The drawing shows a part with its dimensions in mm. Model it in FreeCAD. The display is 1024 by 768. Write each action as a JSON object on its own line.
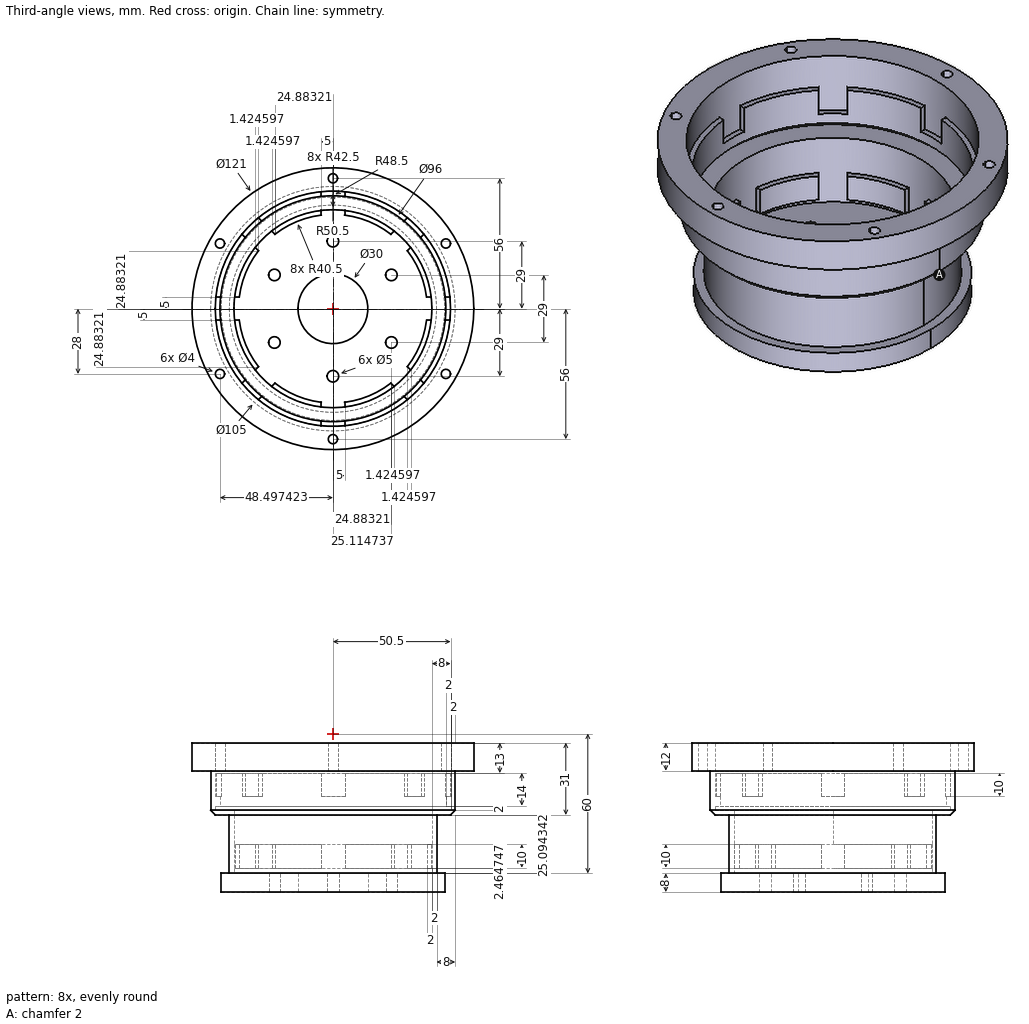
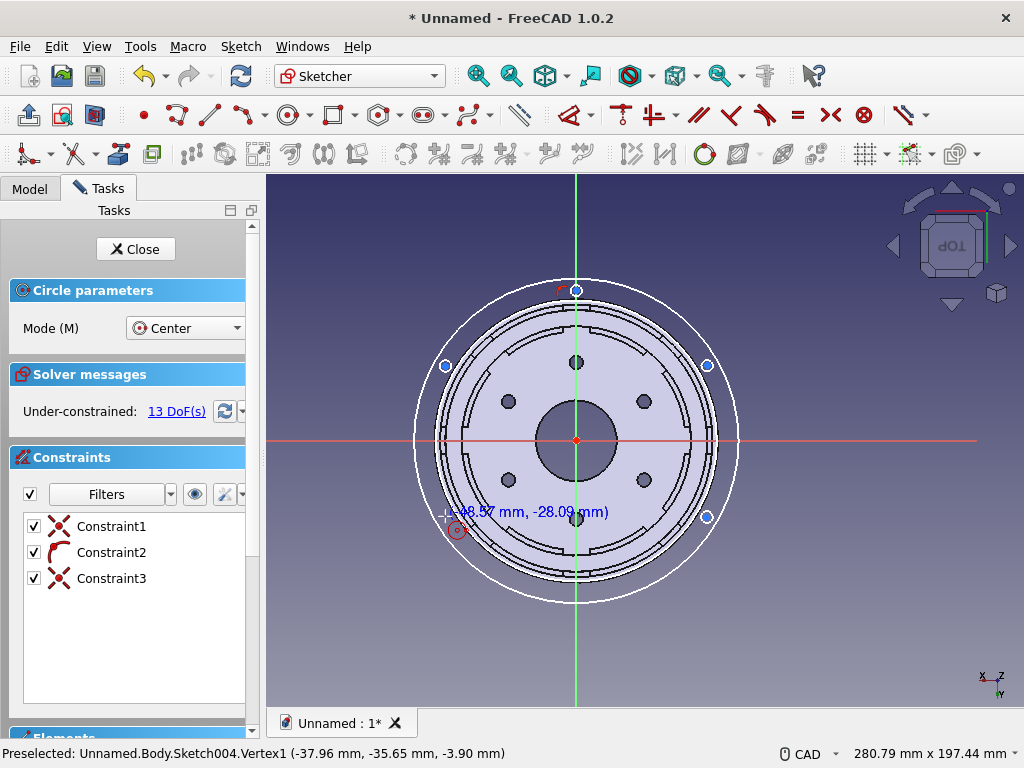
{"action": "scroll", "coordinate": [445, 516], "scroll_direction": "up", "scroll_amount": 3}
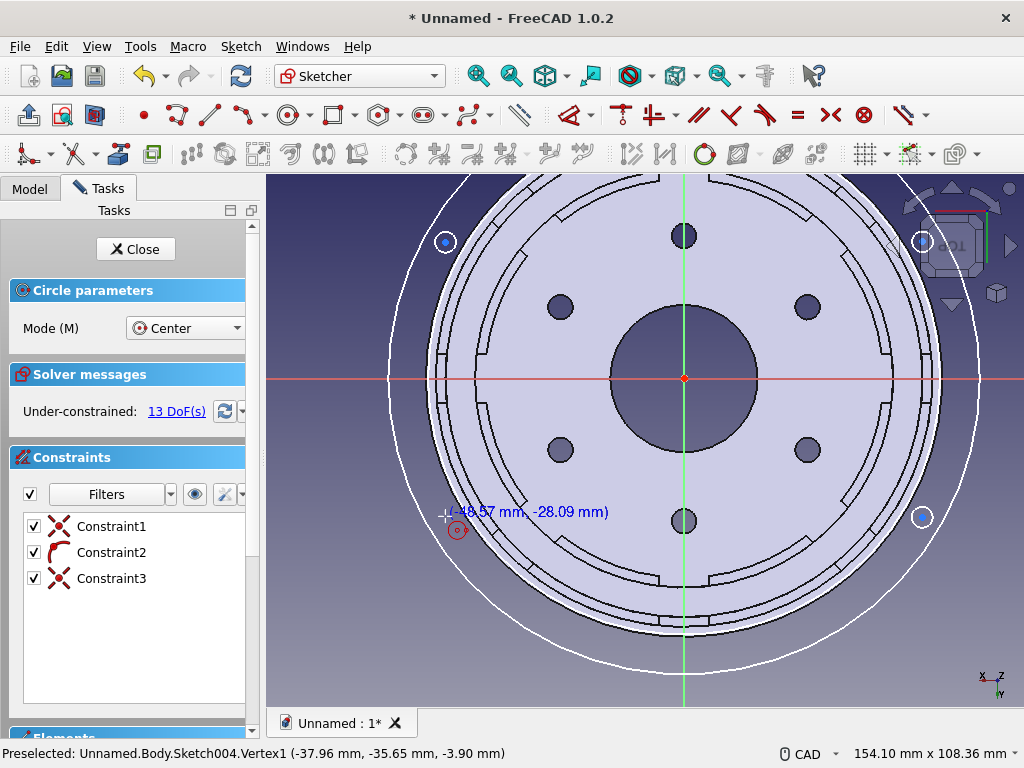
{"action": "left_click", "coordinate": [445, 516]}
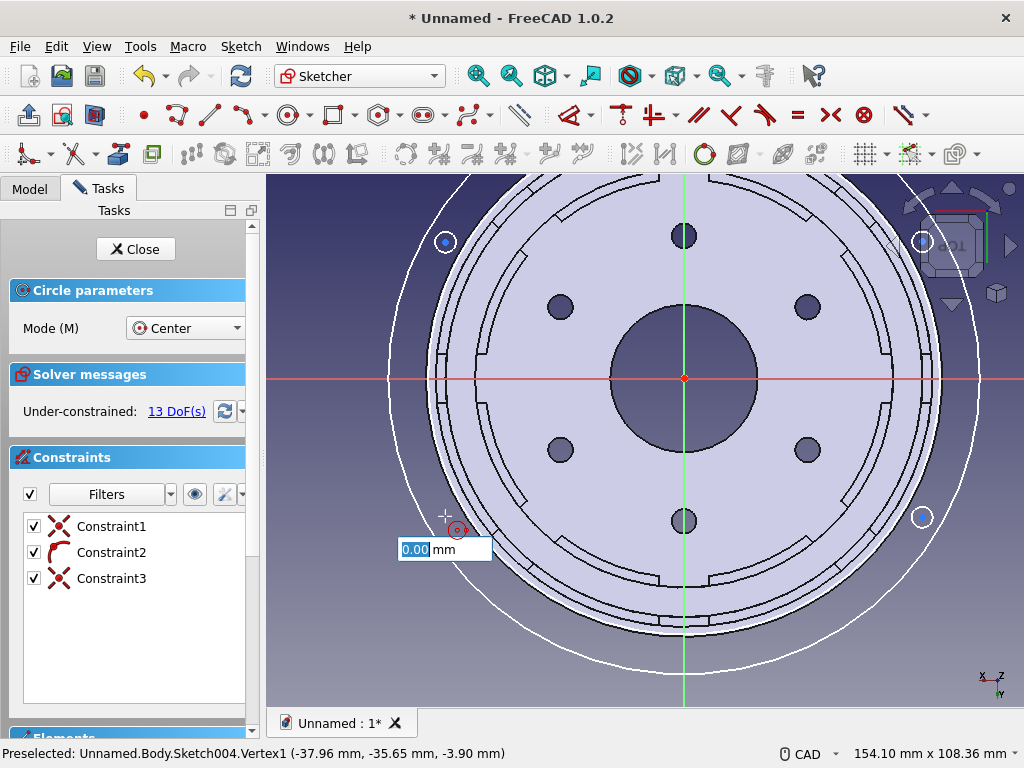
{"action": "scroll", "coordinate": [439, 509], "scroll_direction": "up", "scroll_amount": 3}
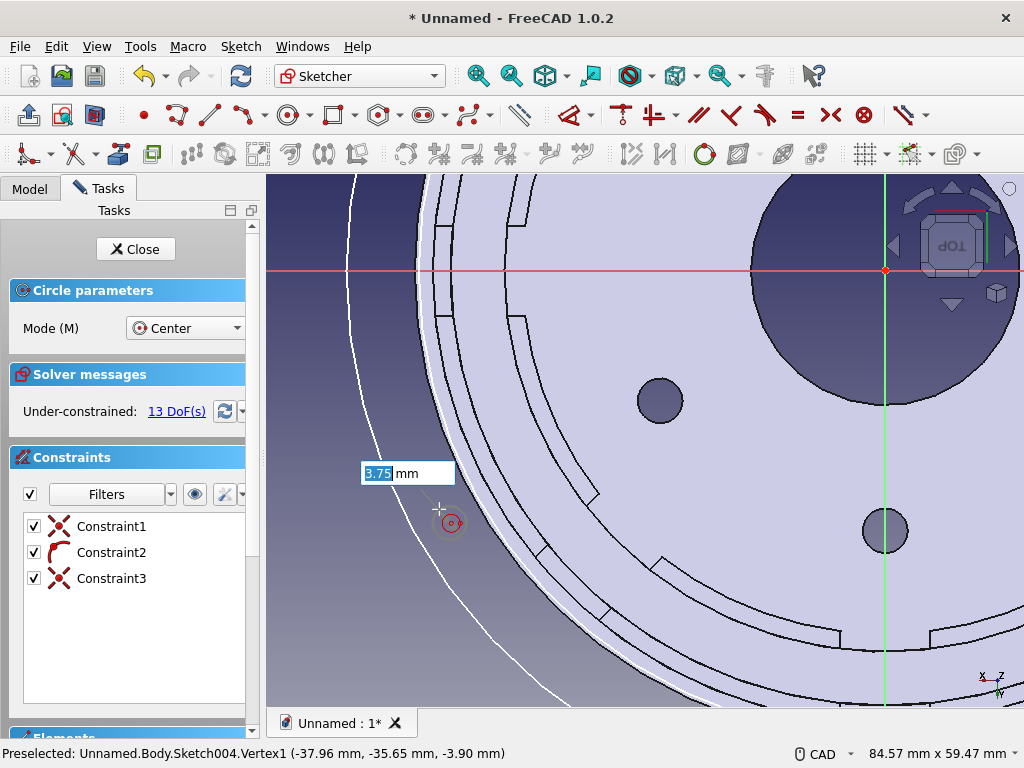
{"action": "left_click", "coordinate": [438, 509]}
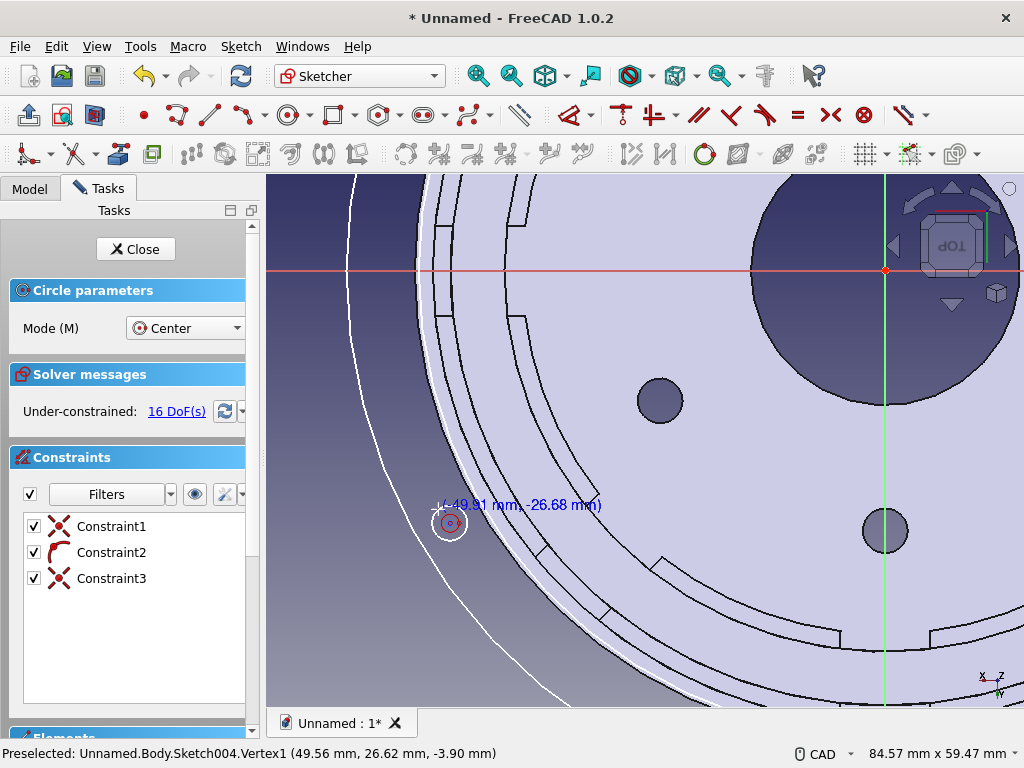
{"action": "scroll", "coordinate": [443, 514], "scroll_direction": "down", "scroll_amount": 6}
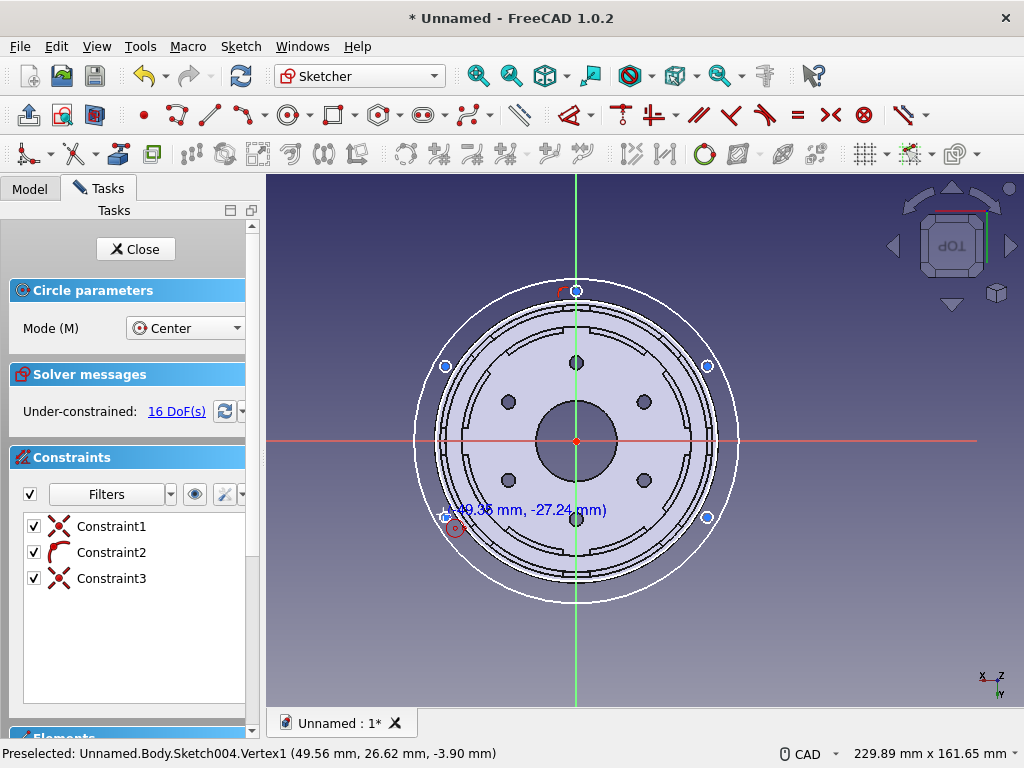
{"action": "scroll", "coordinate": [576, 592], "scroll_direction": "up", "scroll_amount": 8}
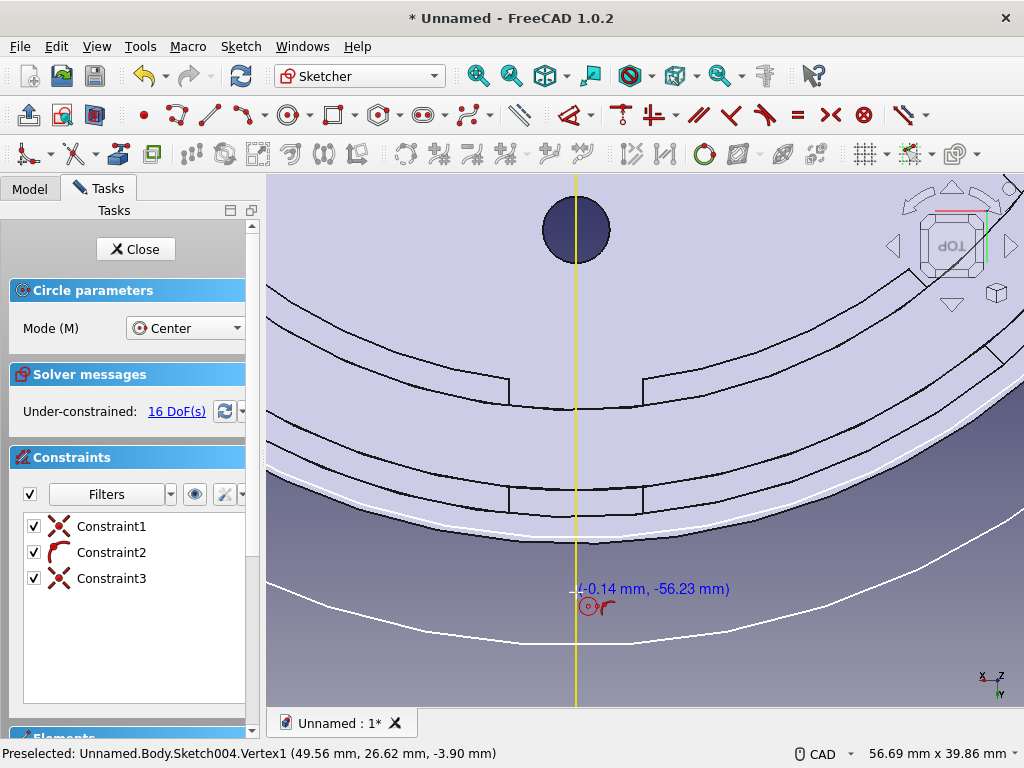
{"action": "scroll", "coordinate": [577, 592], "scroll_direction": "down", "scroll_amount": 8}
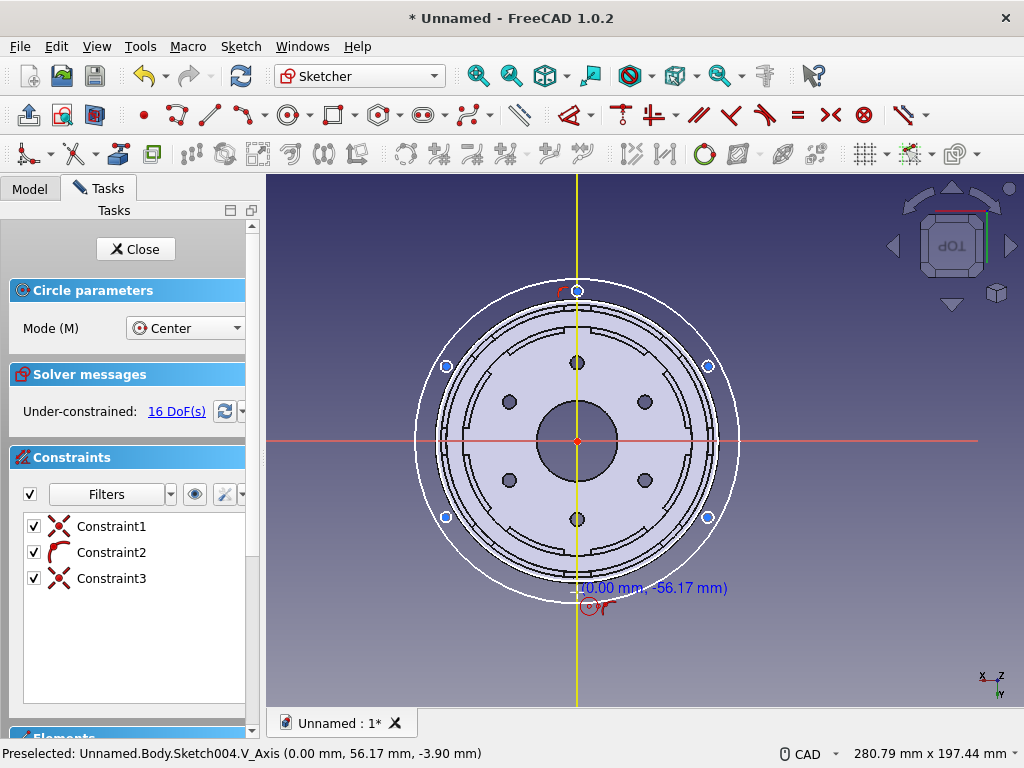
{"action": "scroll", "coordinate": [577, 592], "scroll_direction": "up", "scroll_amount": 3}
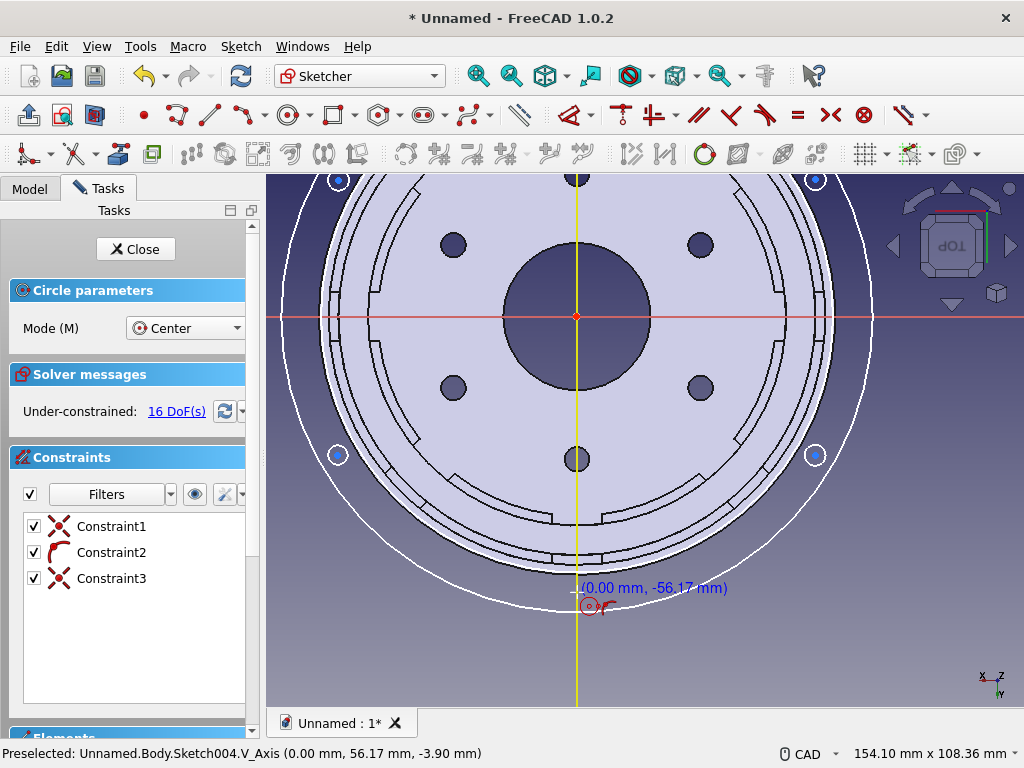
{"action": "left_click", "coordinate": [577, 592]}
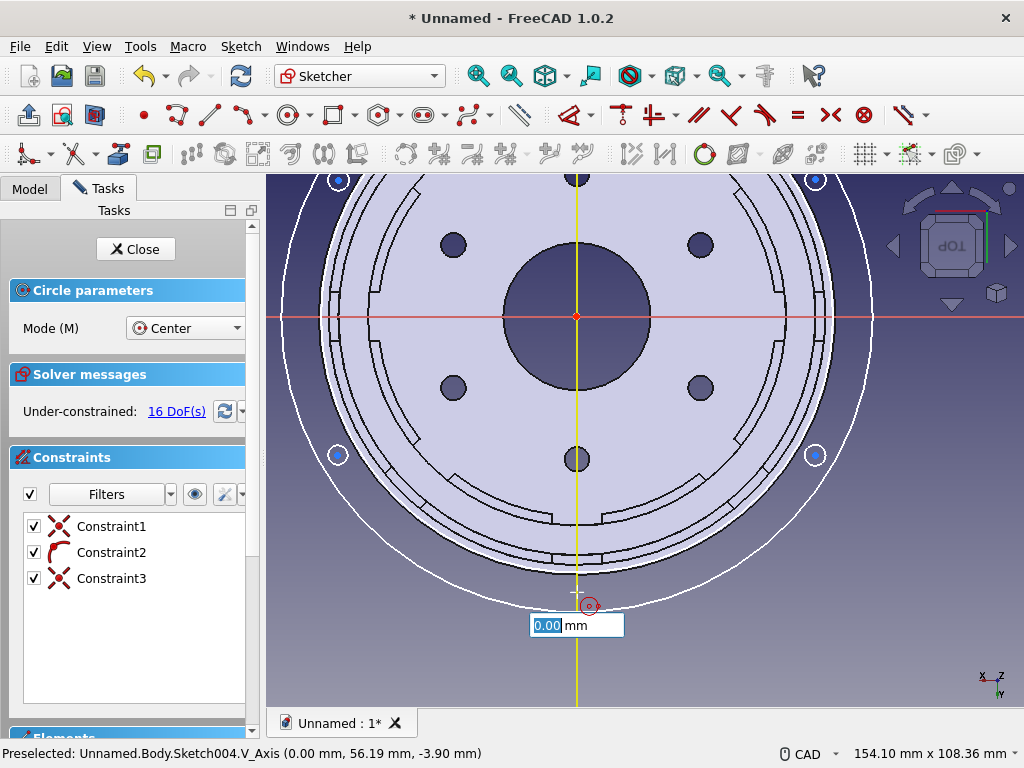
{"action": "scroll", "coordinate": [586, 589], "scroll_direction": "up", "scroll_amount": 3}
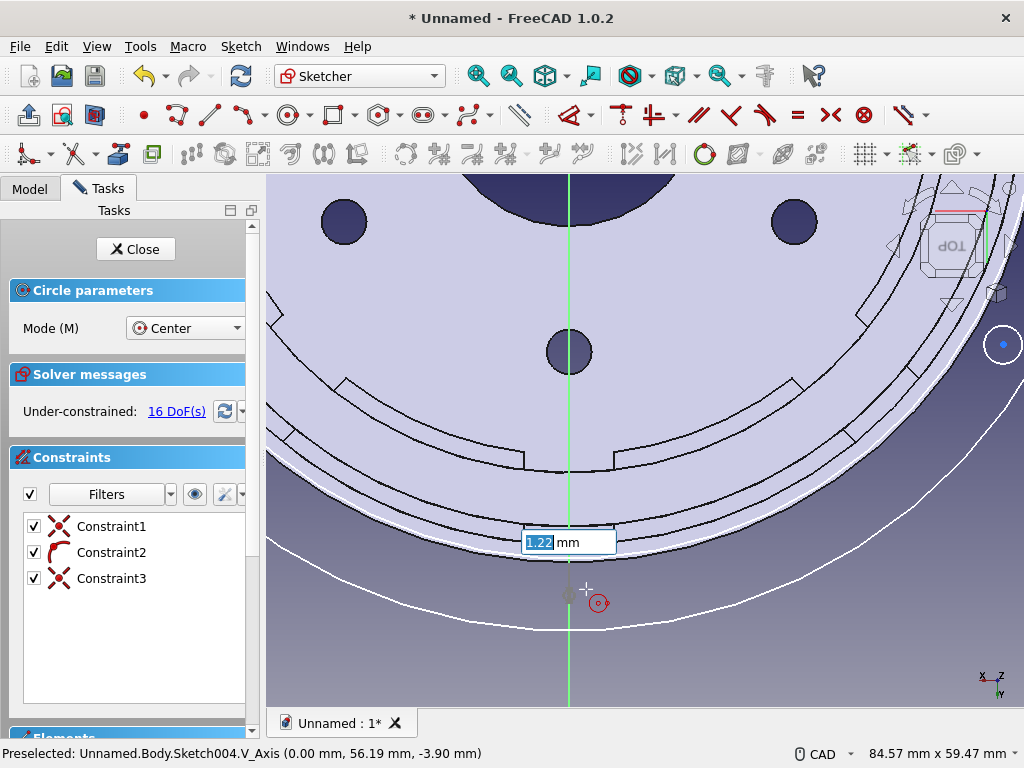
{"action": "left_click", "coordinate": [586, 588]}
{"action": "key", "text": "Escape"}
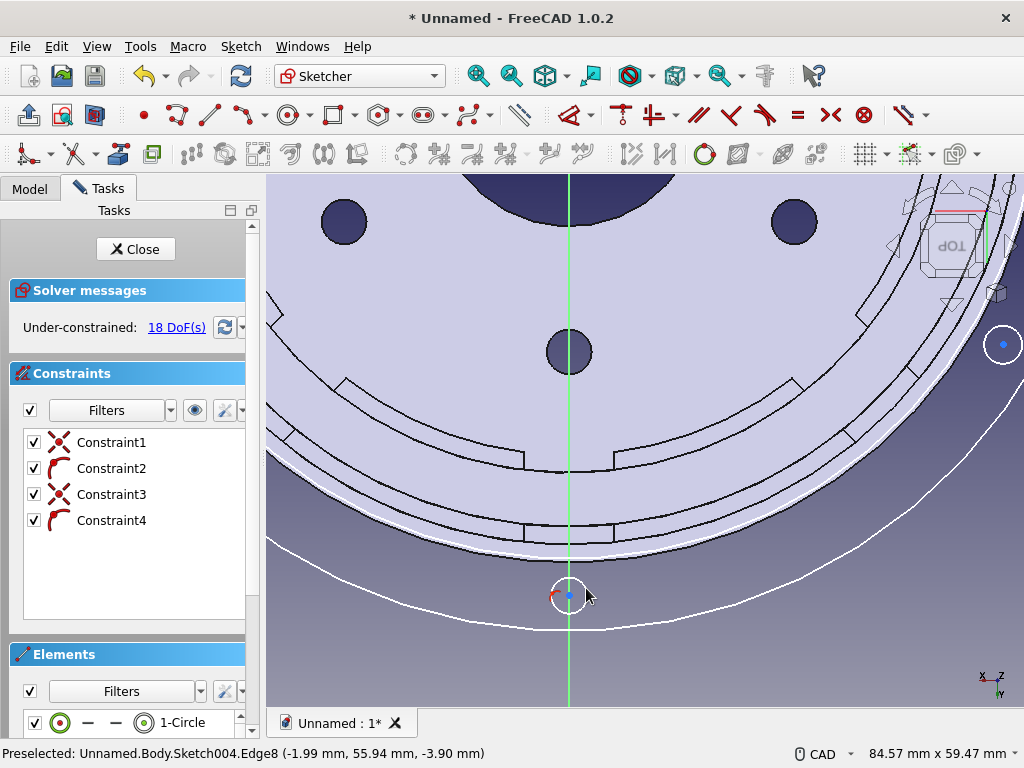
{"action": "scroll", "coordinate": [580, 591], "scroll_direction": "down", "scroll_amount": 6}